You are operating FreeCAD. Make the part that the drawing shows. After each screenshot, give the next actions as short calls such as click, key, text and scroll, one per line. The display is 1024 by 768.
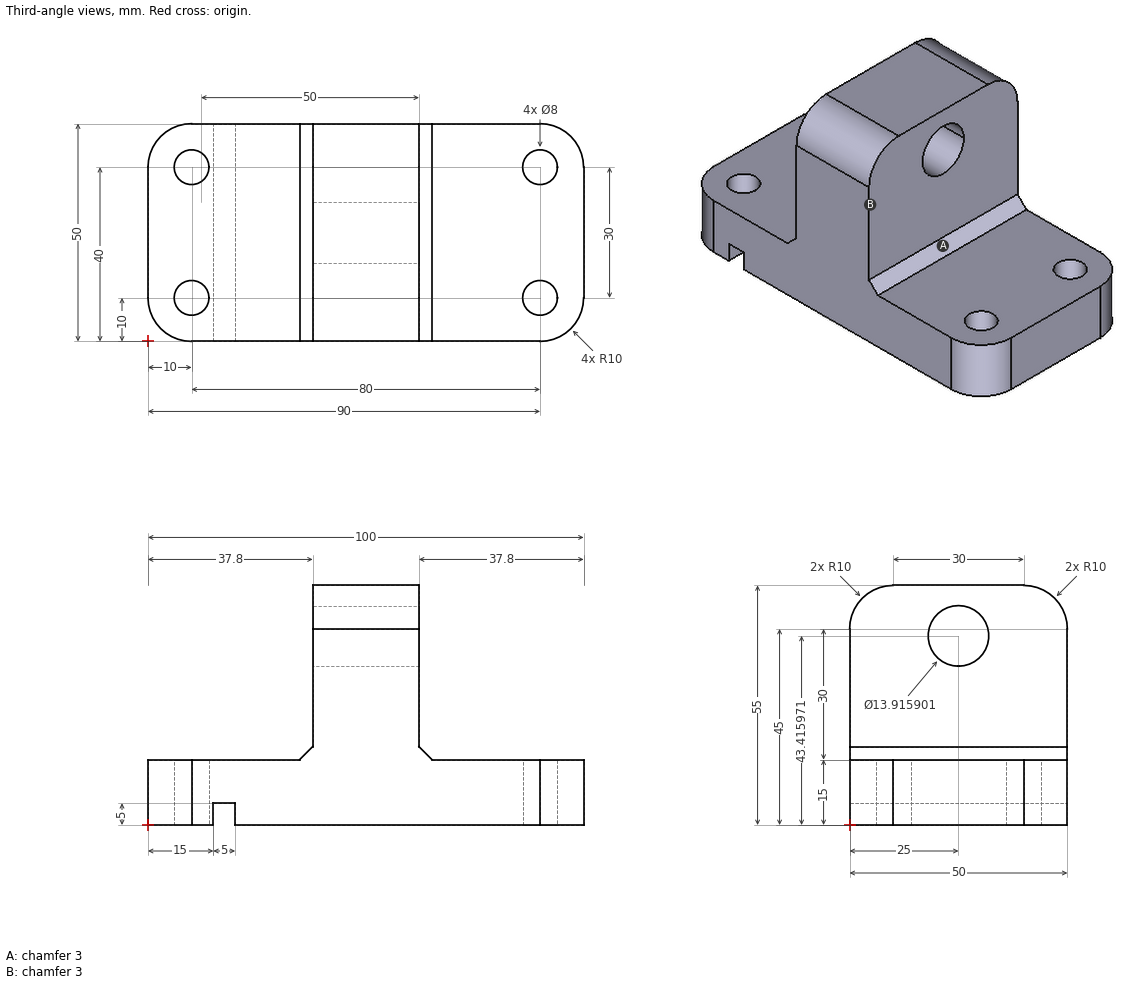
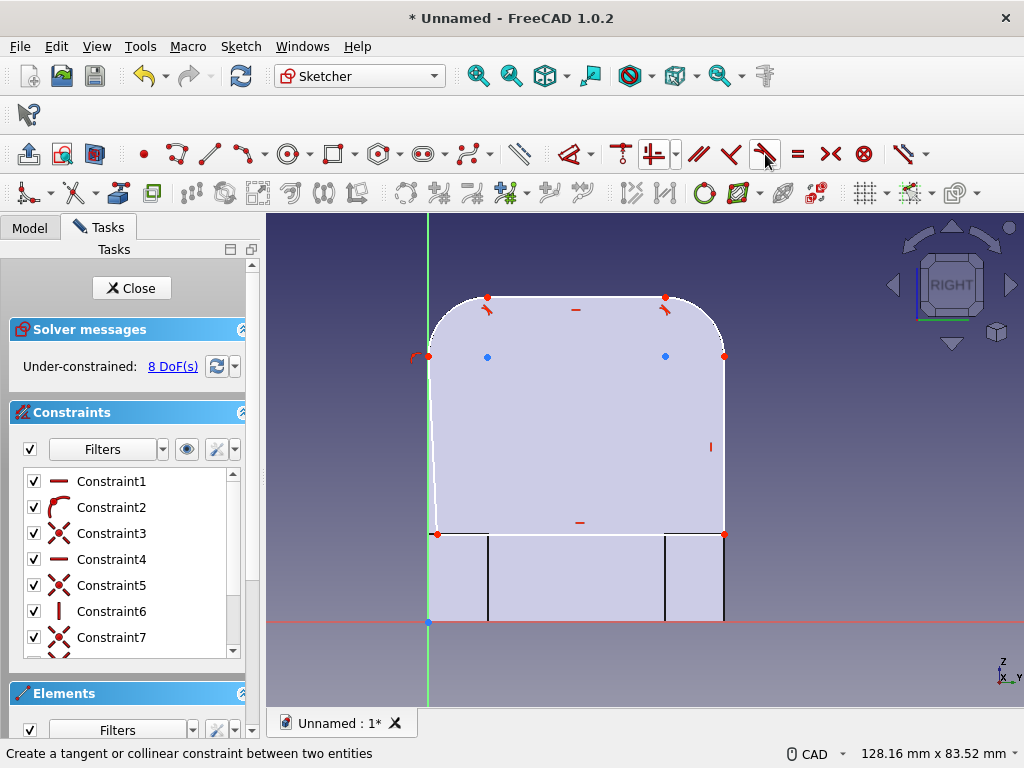
click(431, 410)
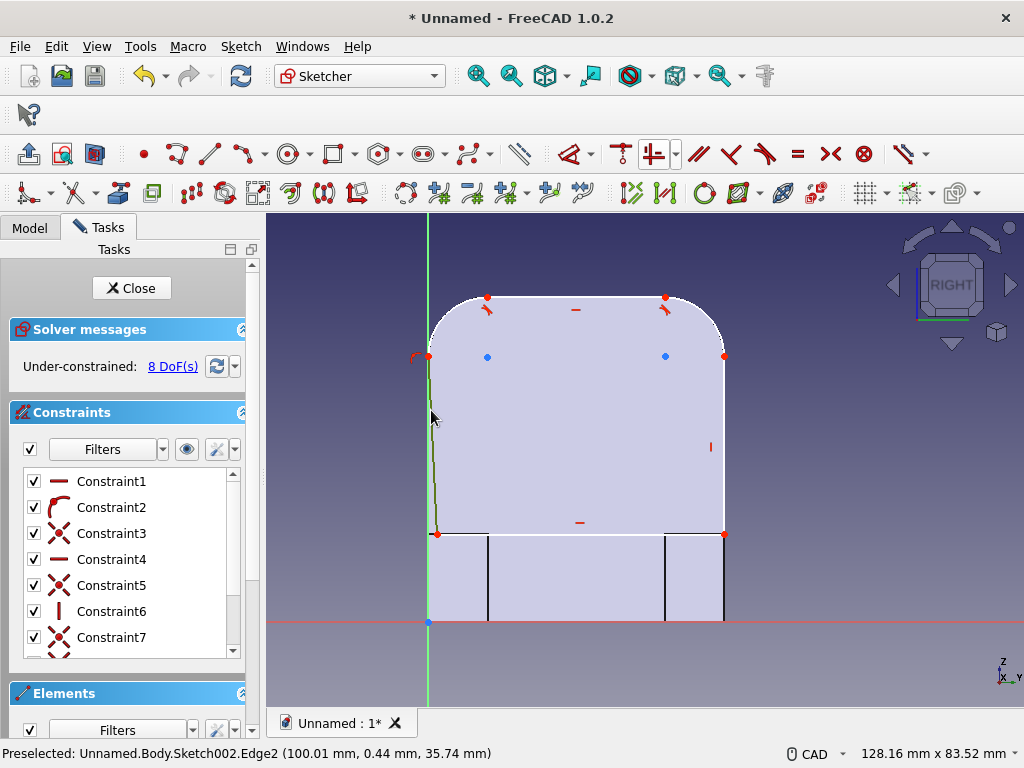
click(461, 304)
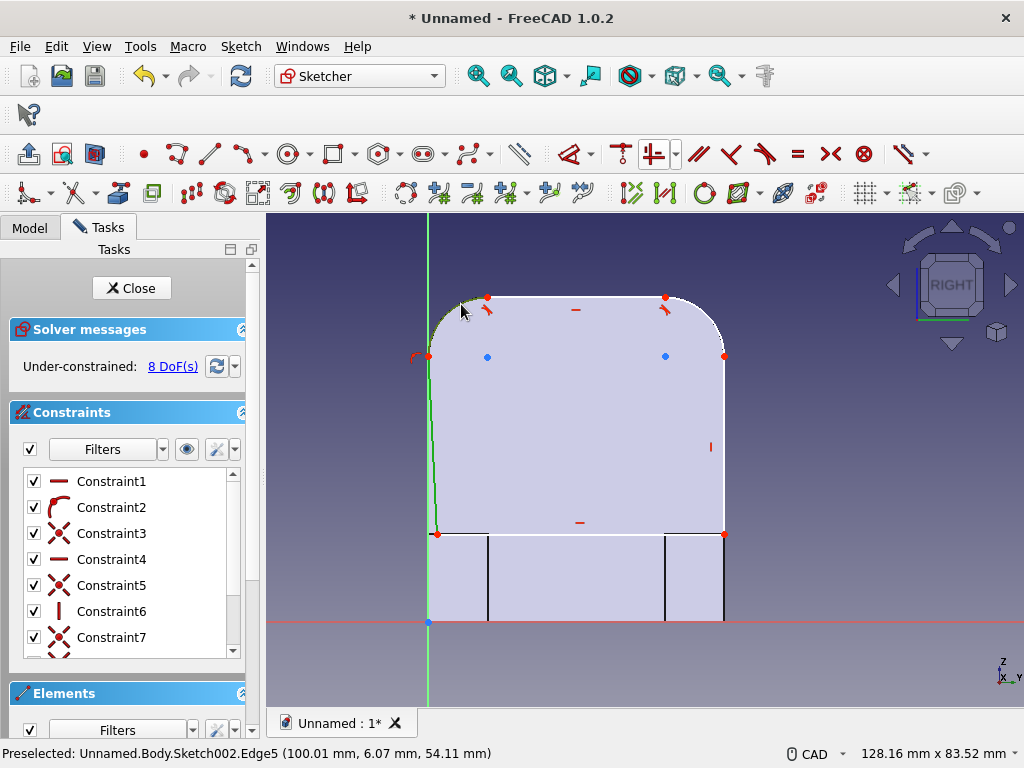
click(765, 154)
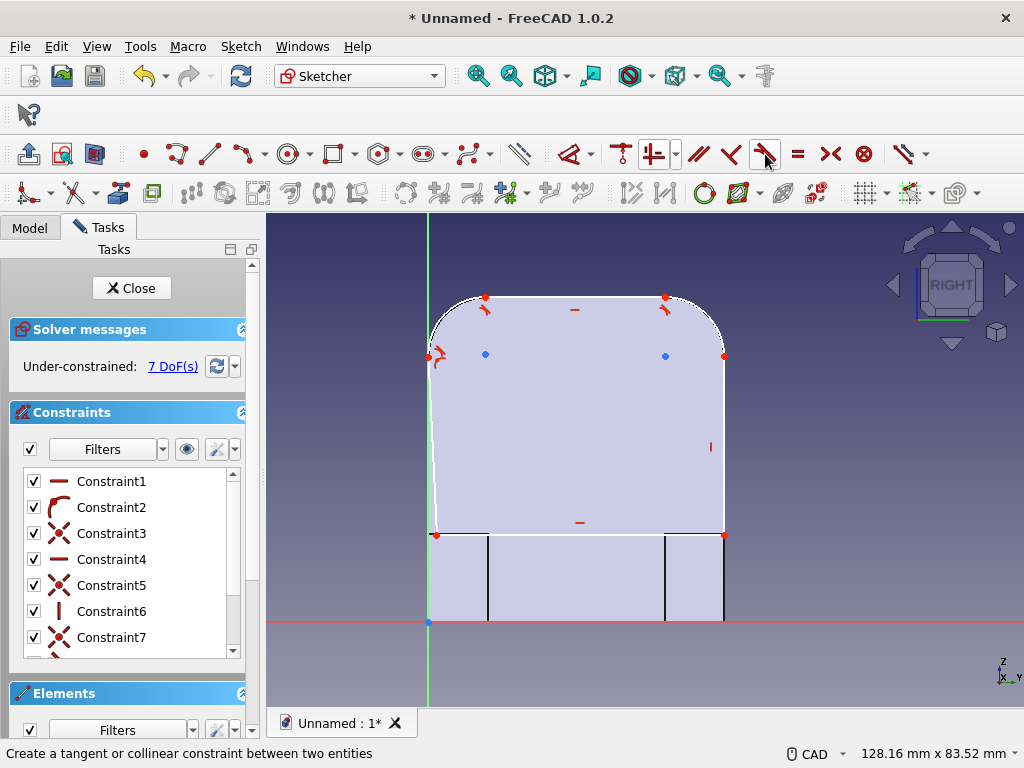
click(724, 482)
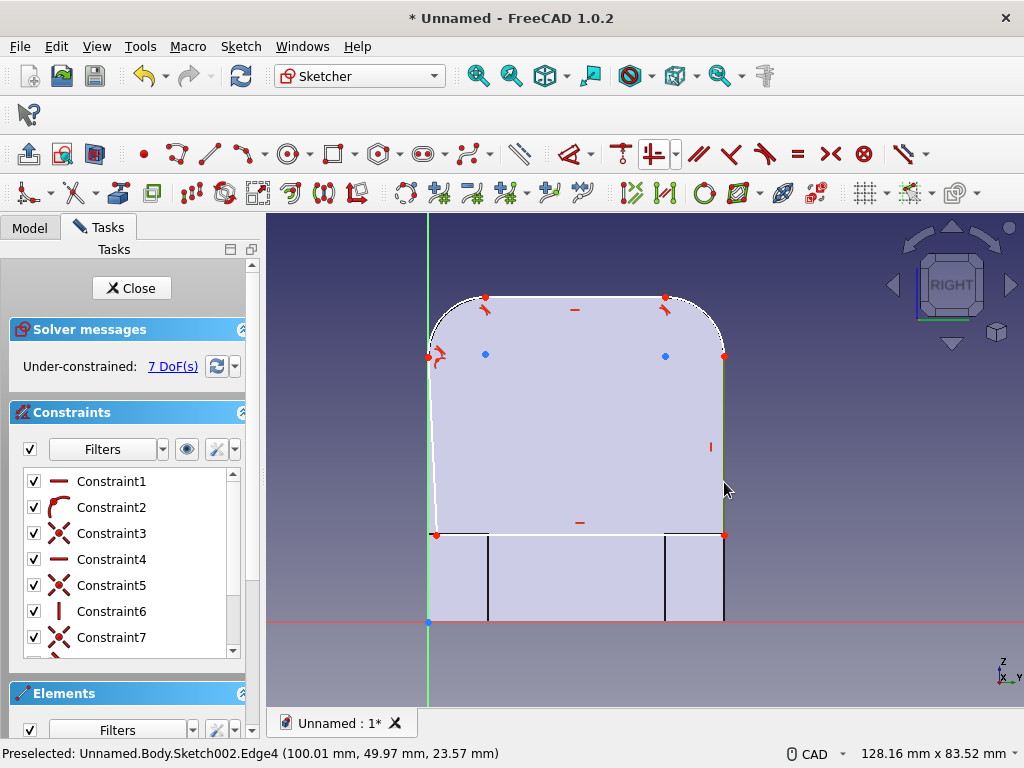
click(718, 330)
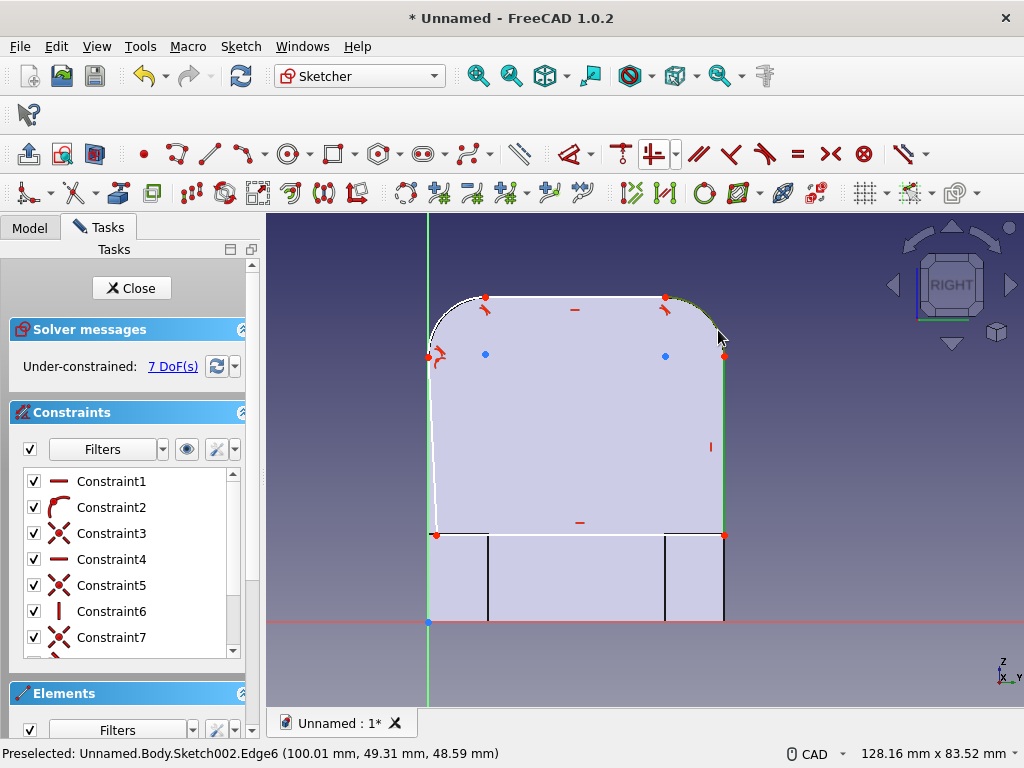
click(765, 154)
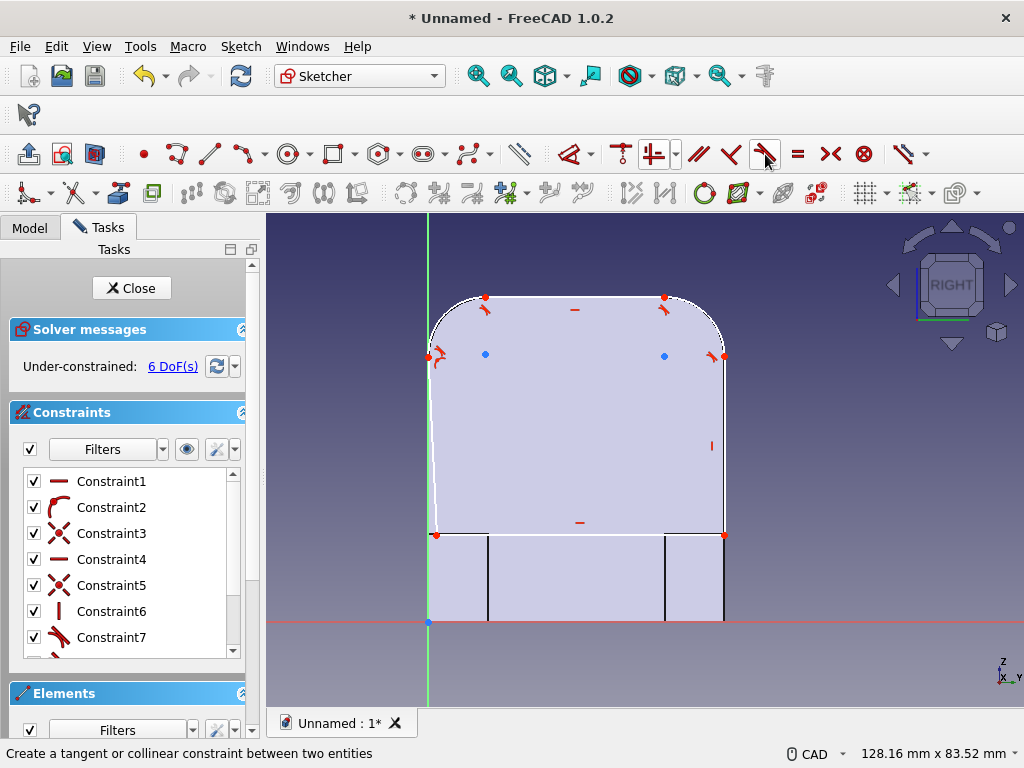
click(431, 410)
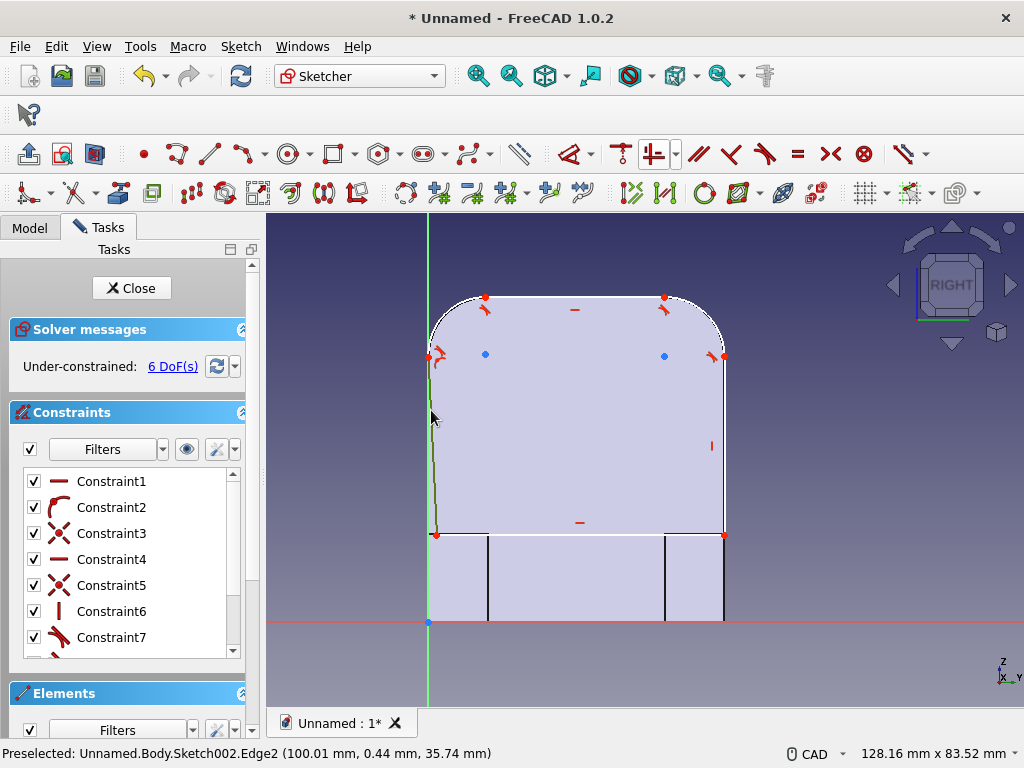
click(676, 154)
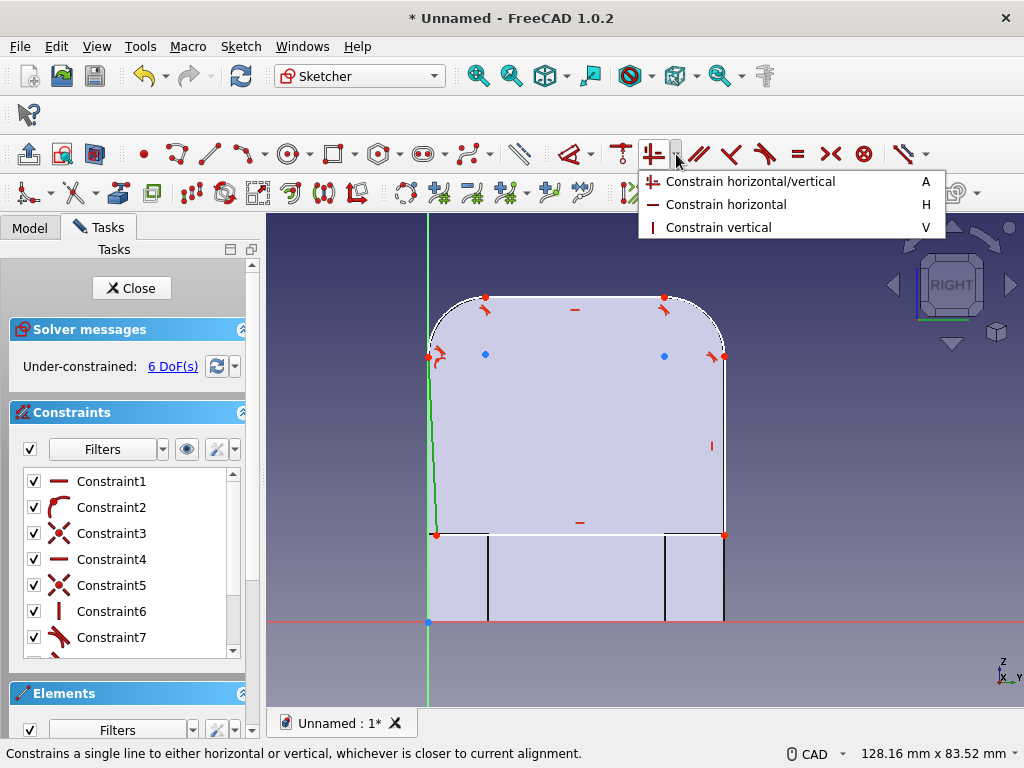
click(792, 228)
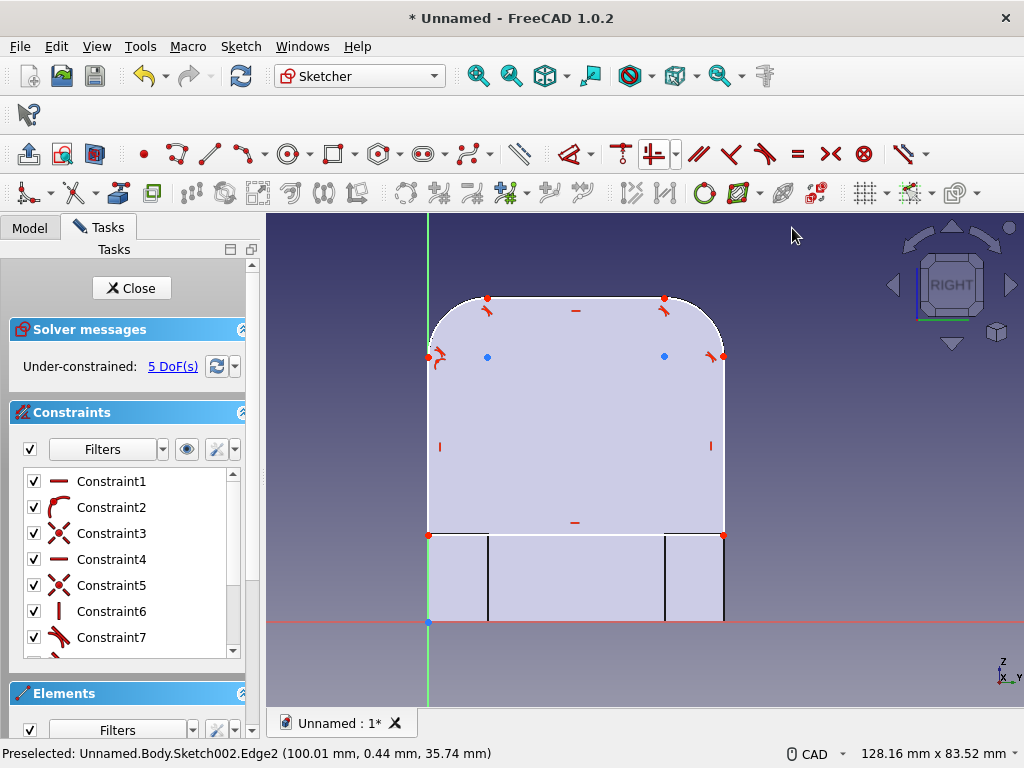
click(461, 305)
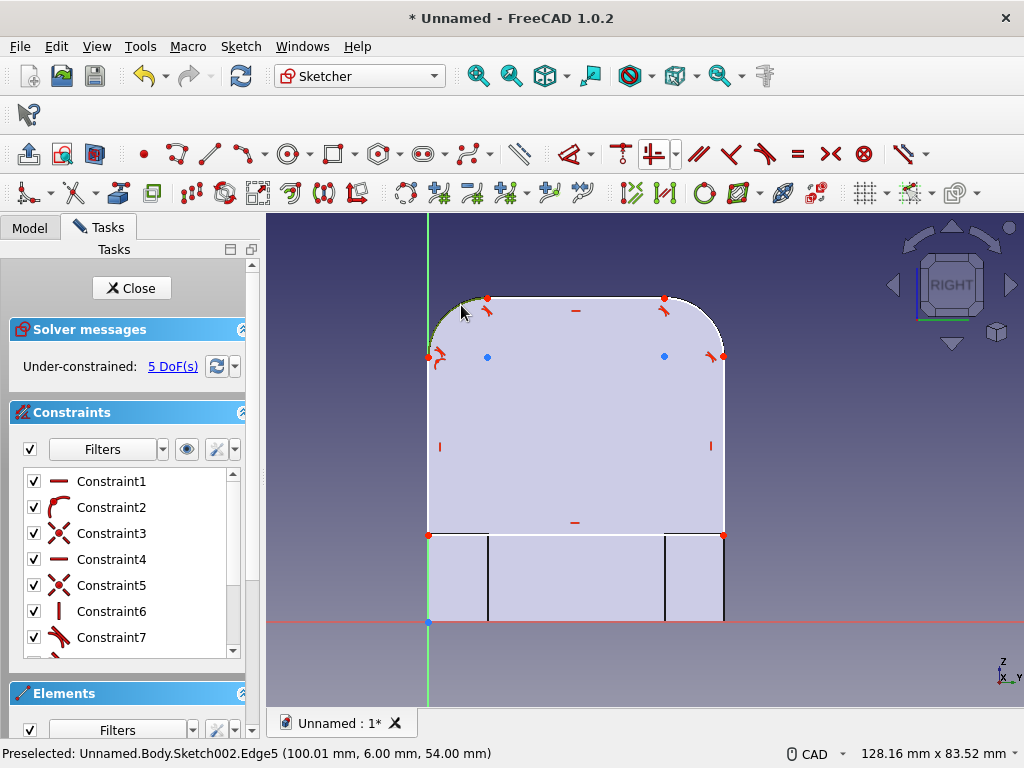
click(717, 330)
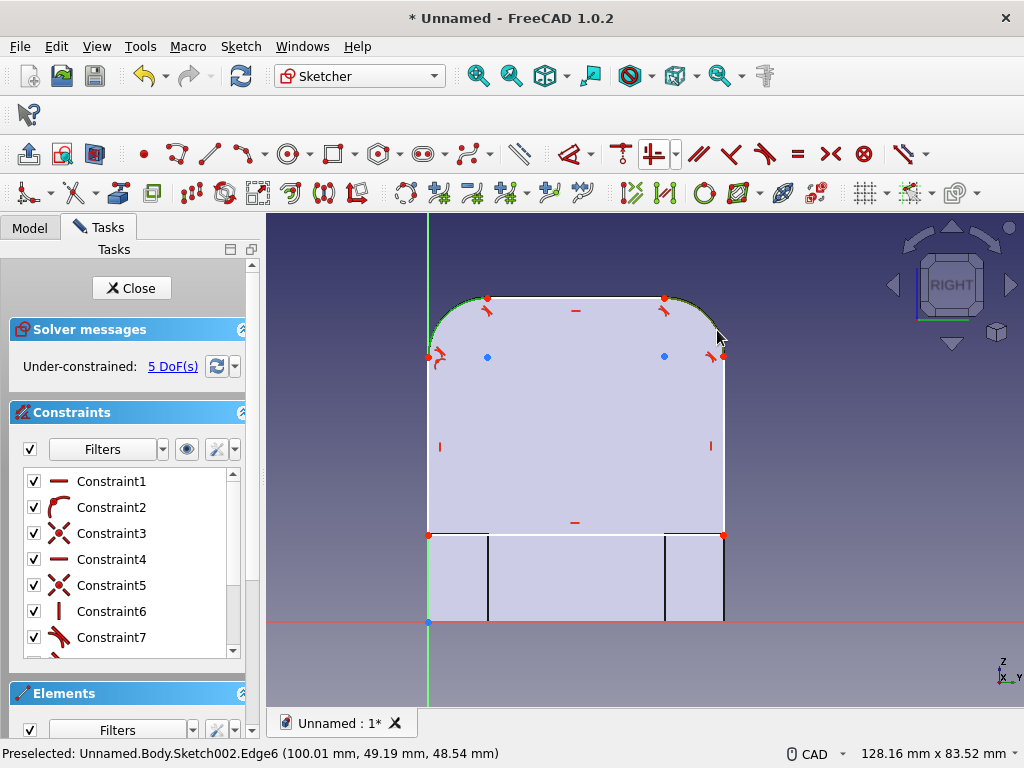
click(798, 154)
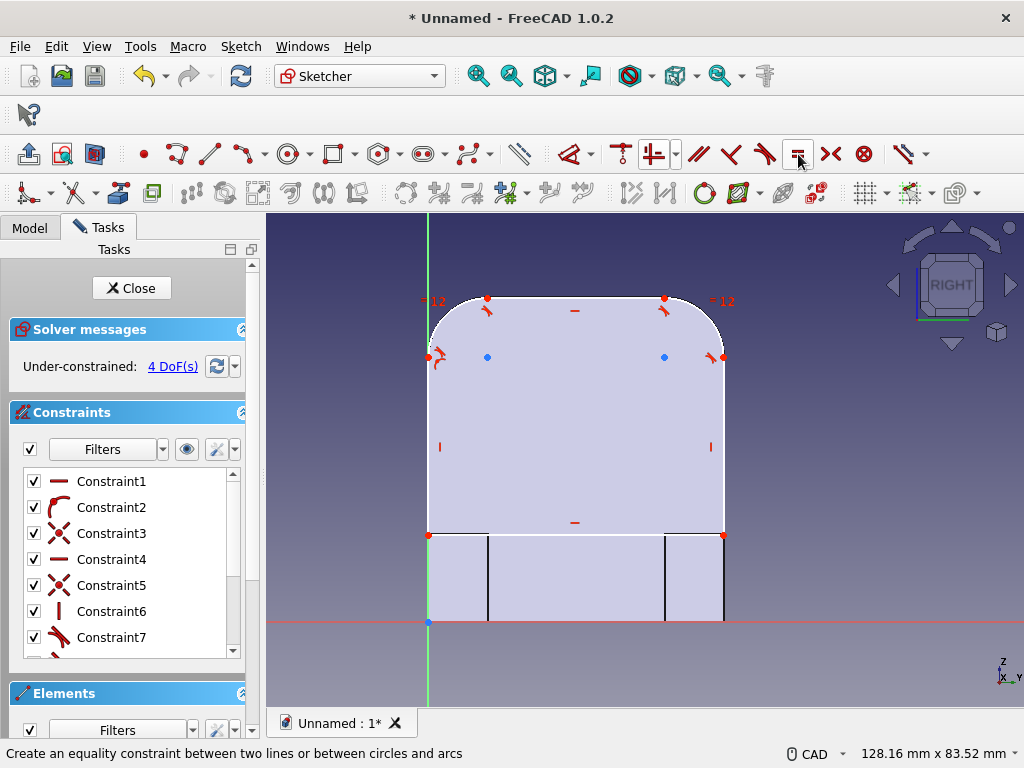
click(568, 154)